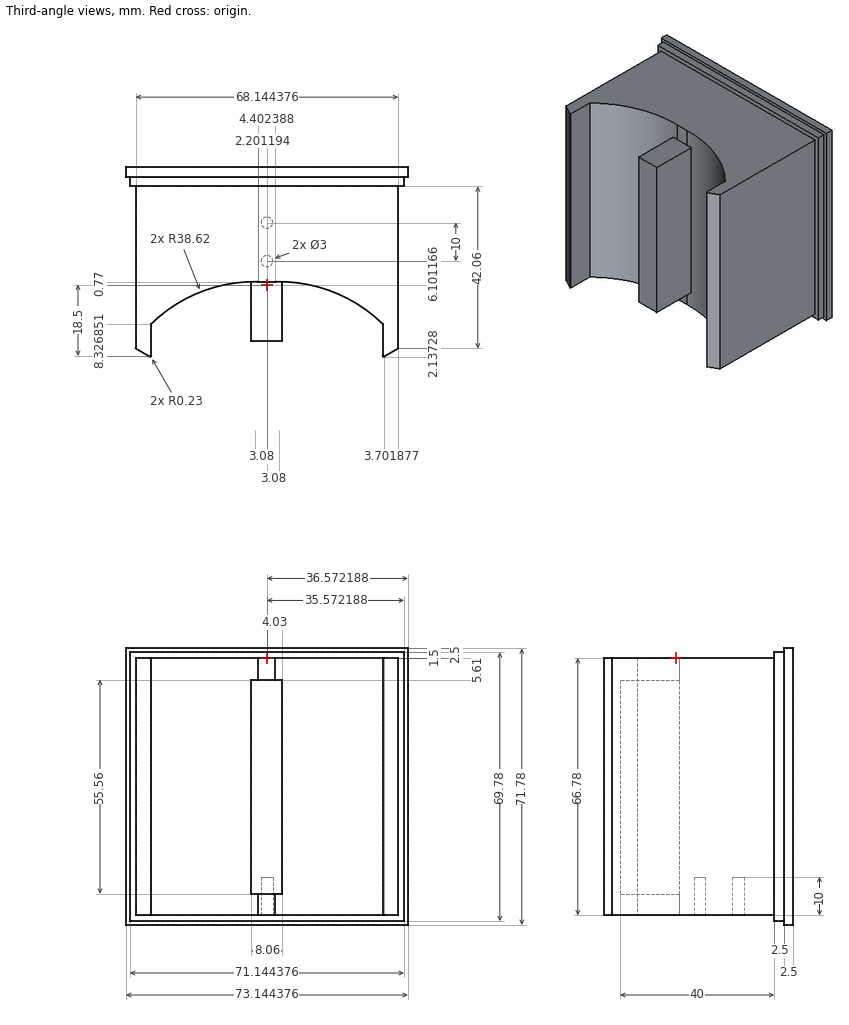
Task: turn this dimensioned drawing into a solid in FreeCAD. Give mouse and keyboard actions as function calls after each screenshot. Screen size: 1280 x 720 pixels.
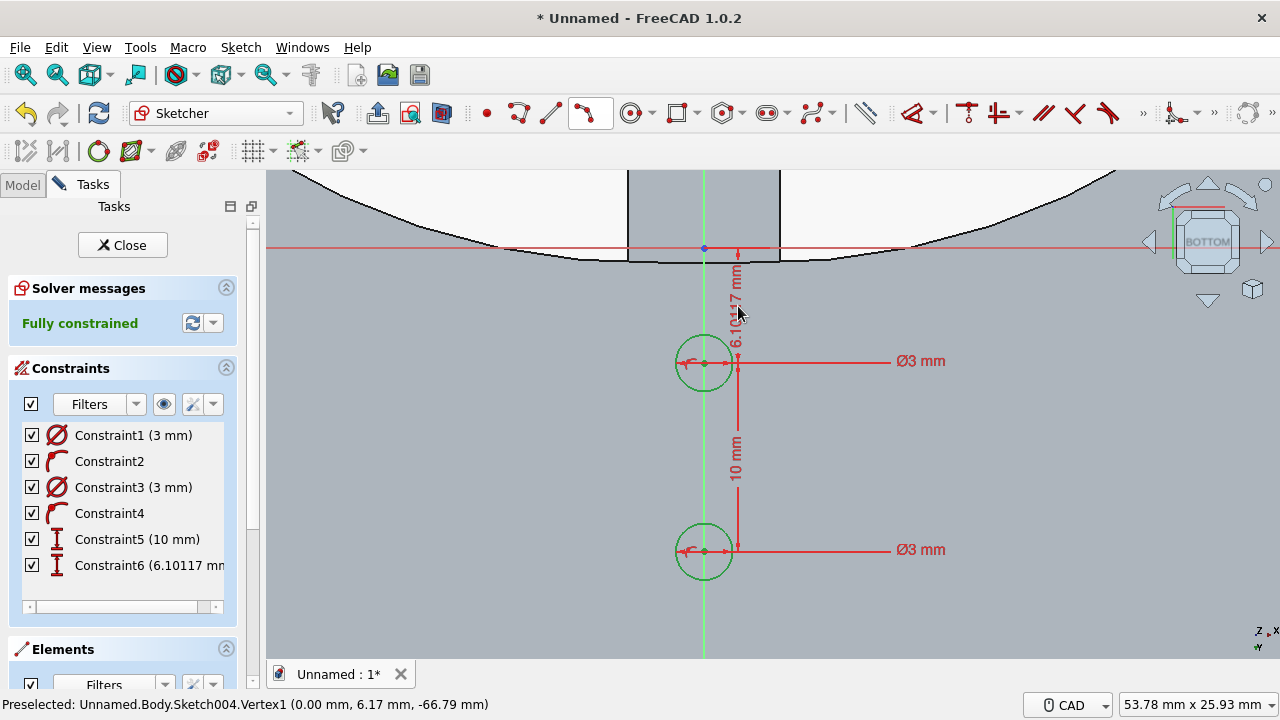
click(123, 245)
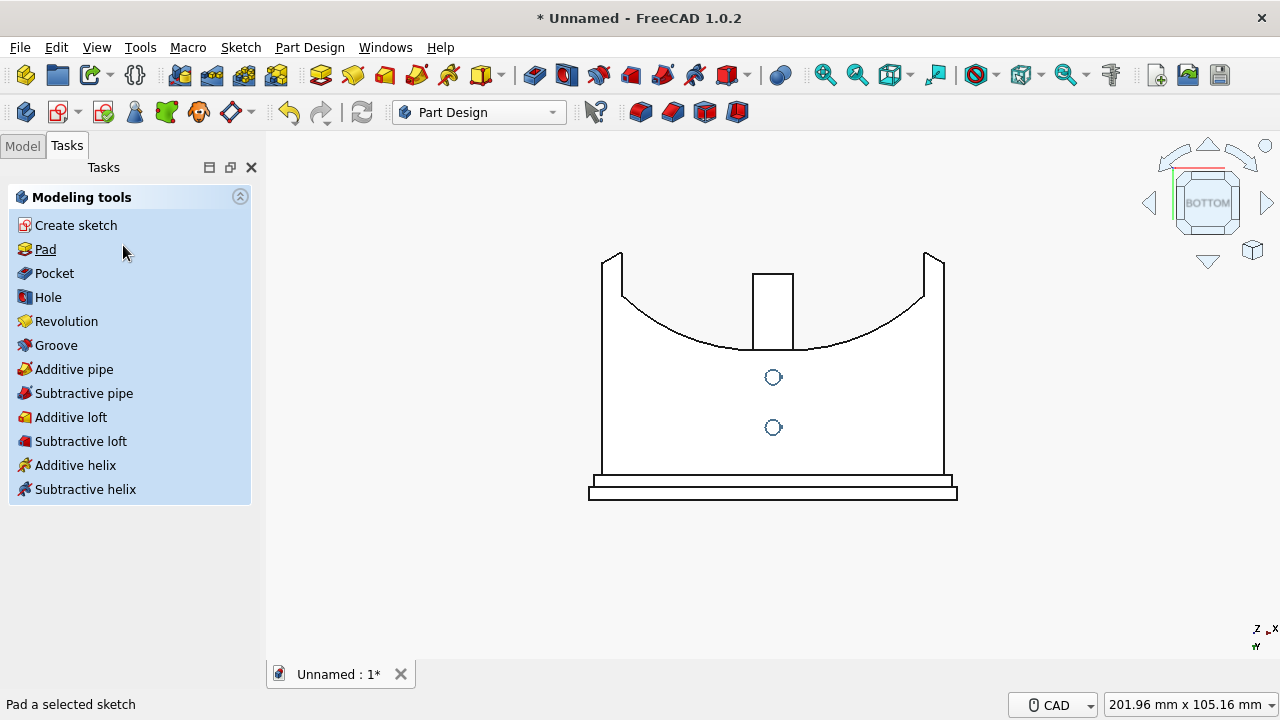
click(536, 76)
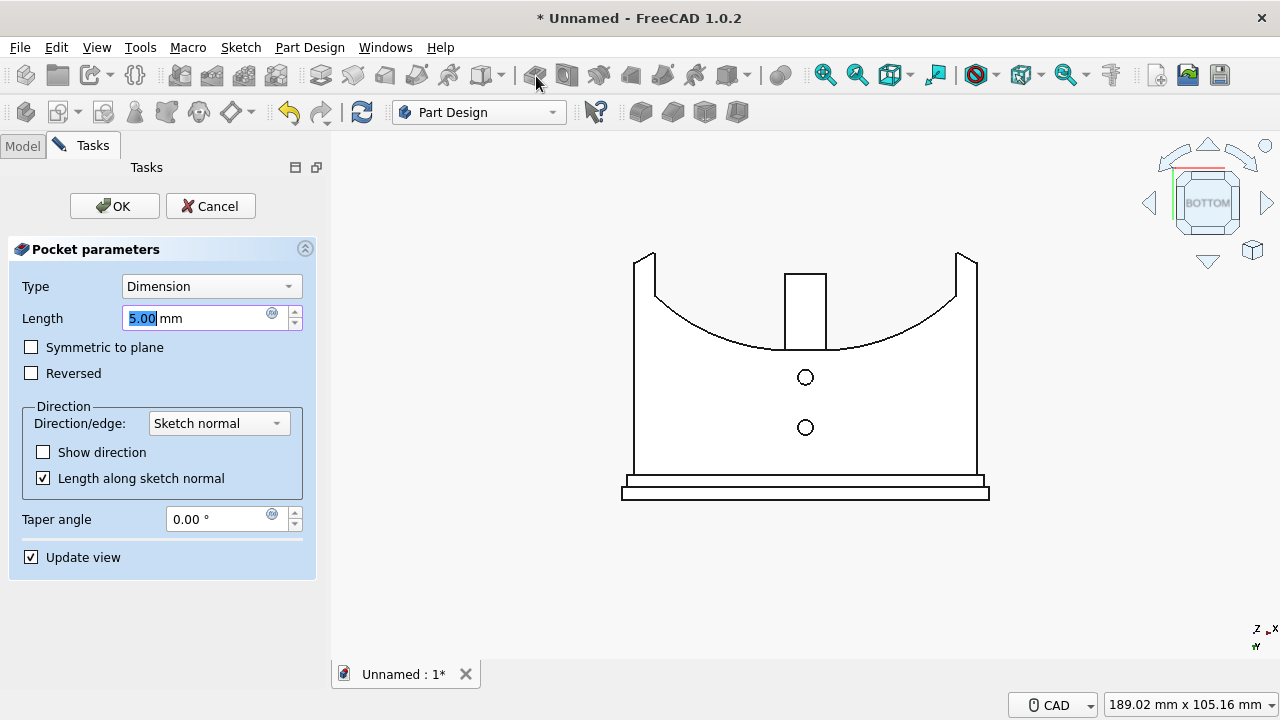
text(10)
key(Tab)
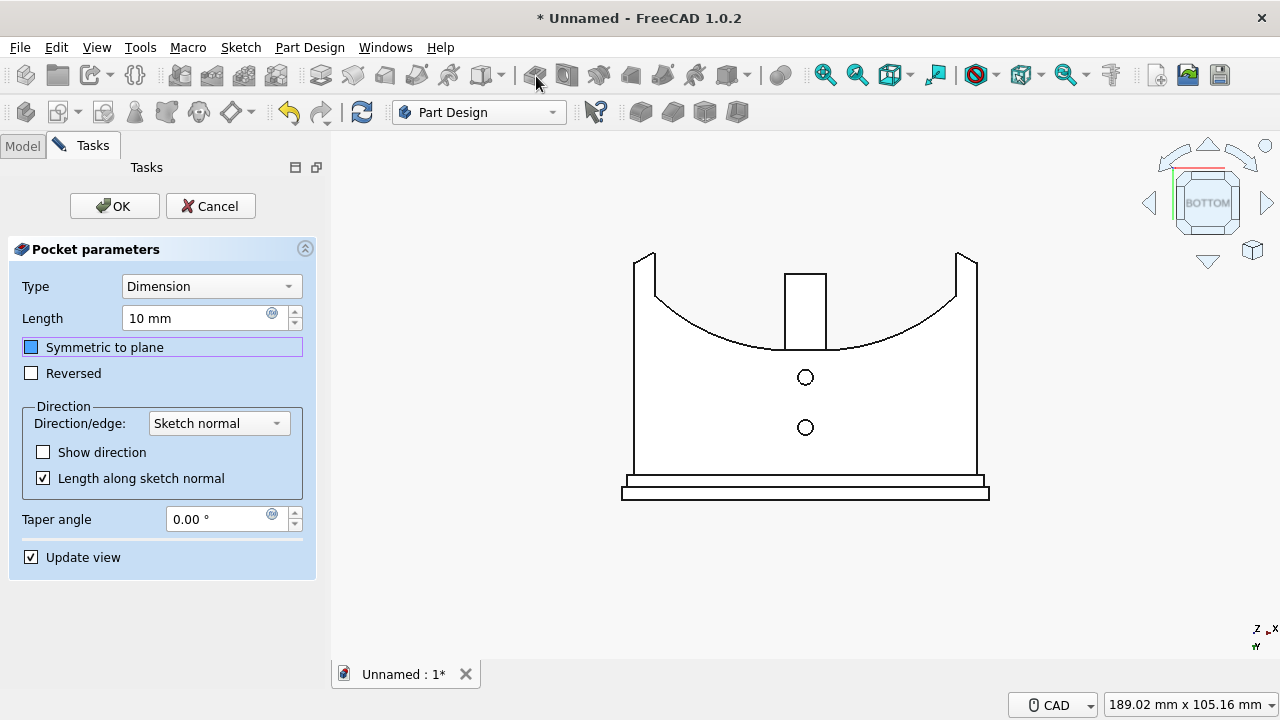
click(115, 206)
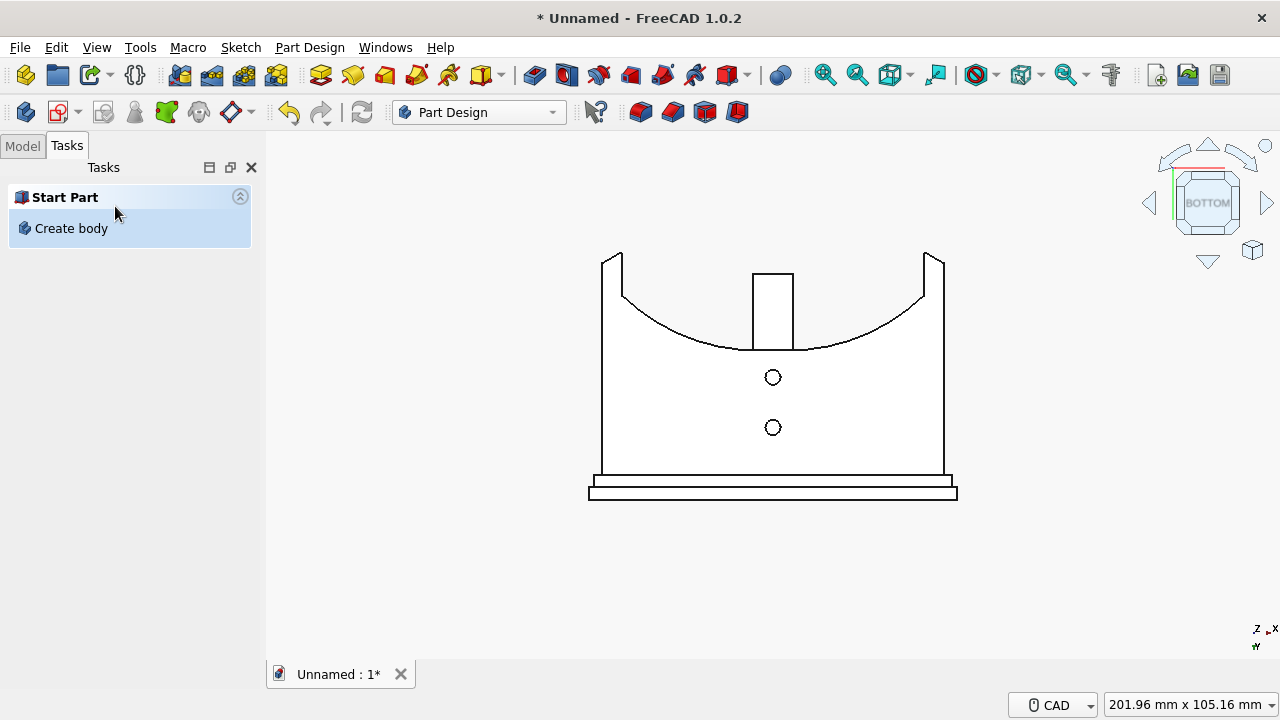
key(0)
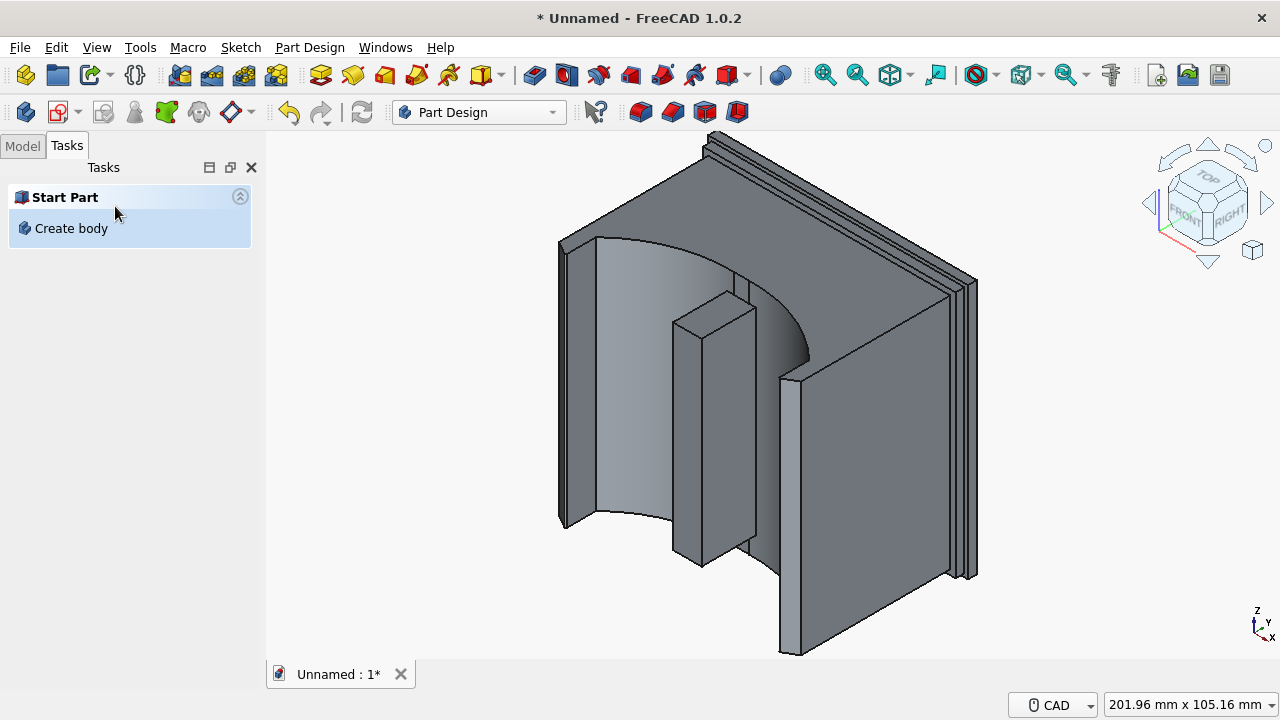
click(826, 76)